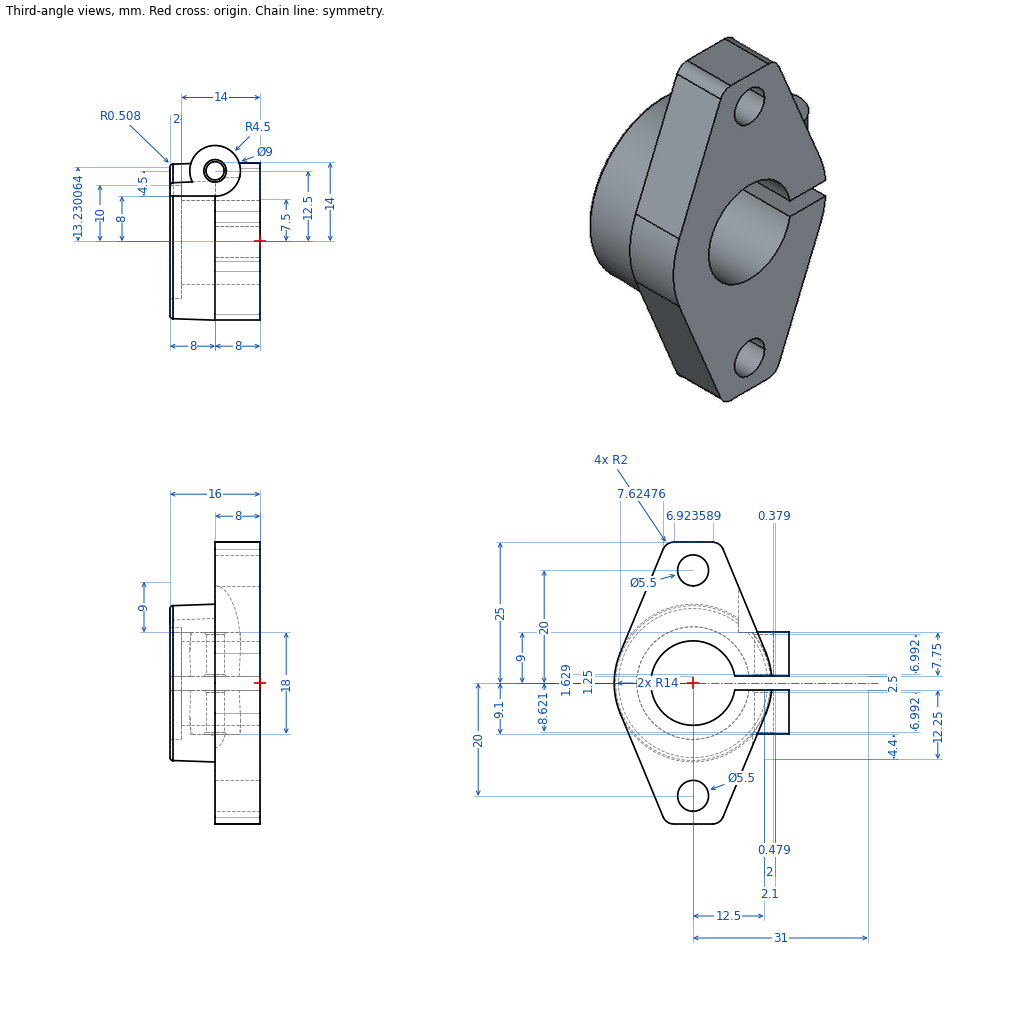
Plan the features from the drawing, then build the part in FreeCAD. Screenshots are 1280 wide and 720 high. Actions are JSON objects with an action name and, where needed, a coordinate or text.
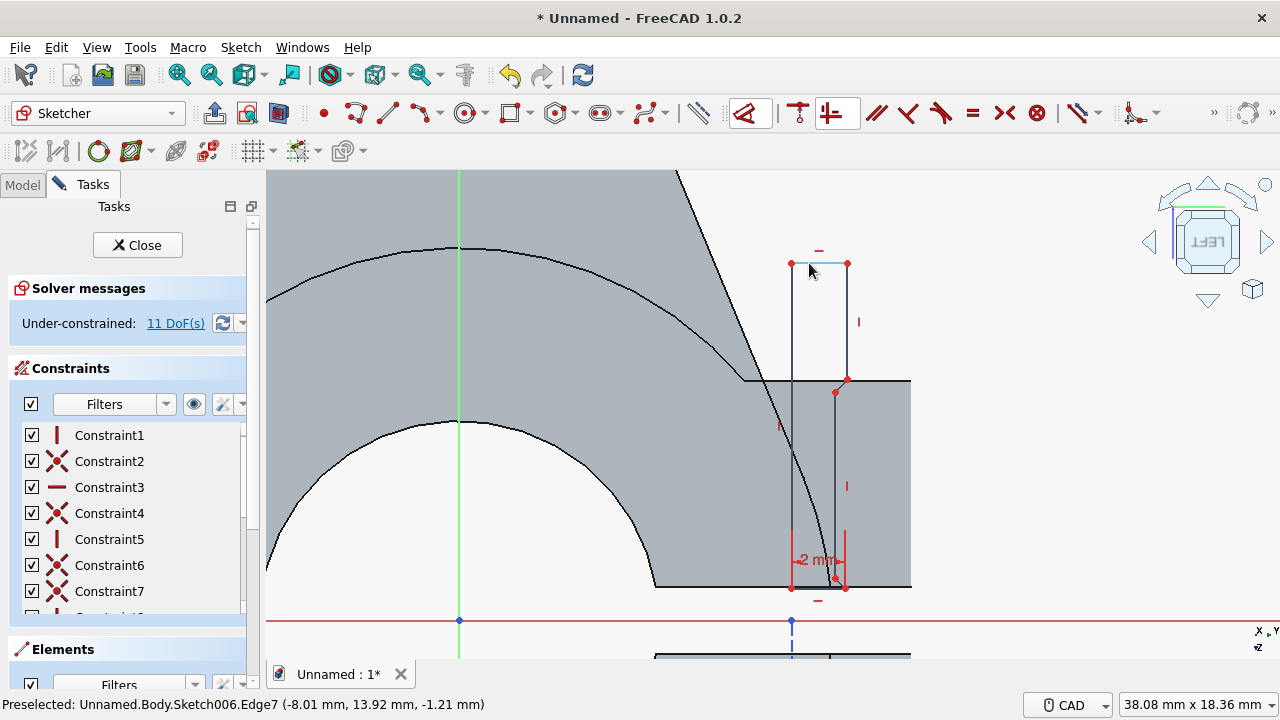
{"action": "left_click", "coordinate": [809, 263]}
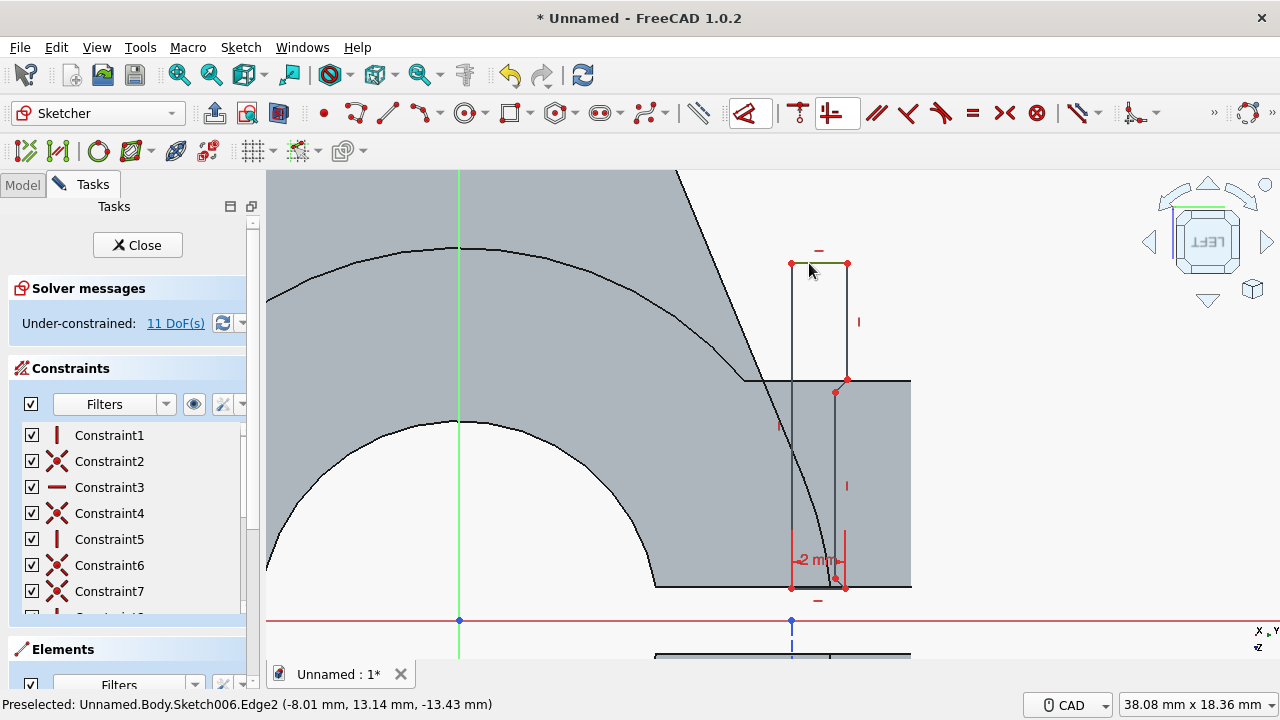
{"action": "key", "text": "l"}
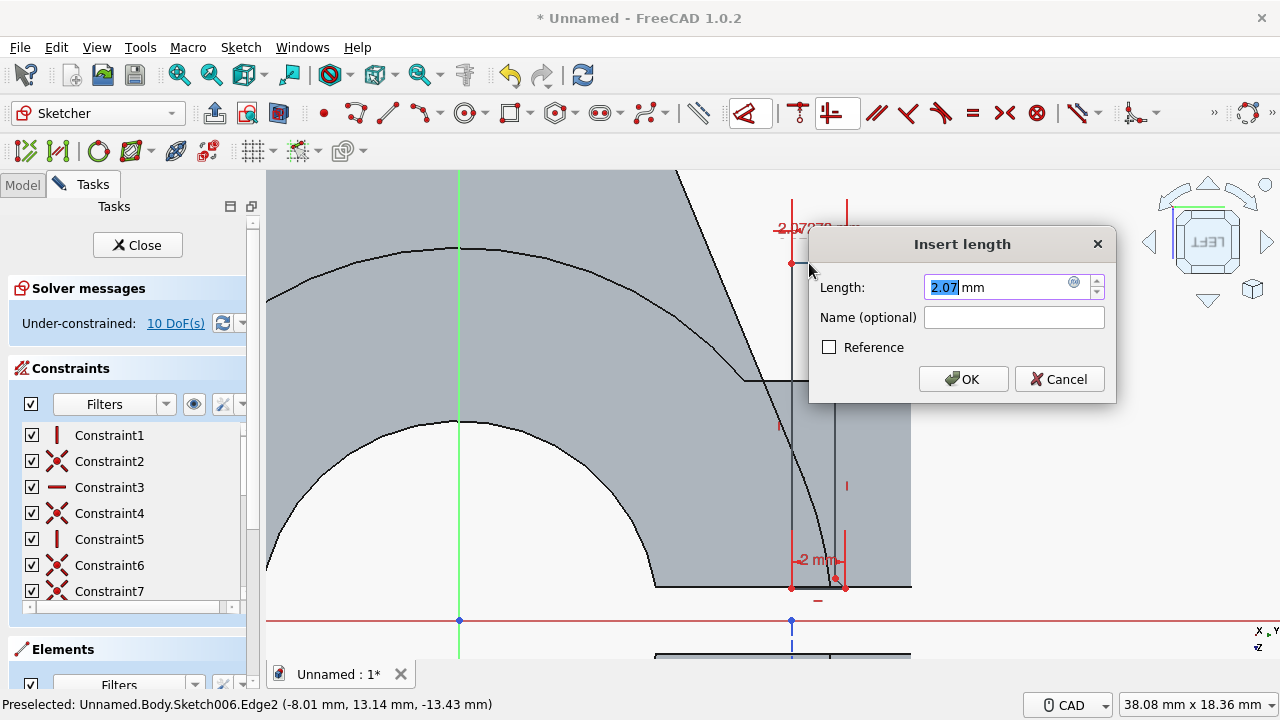
{"action": "type", "text": "2.1"}
{"action": "key", "text": "Return"}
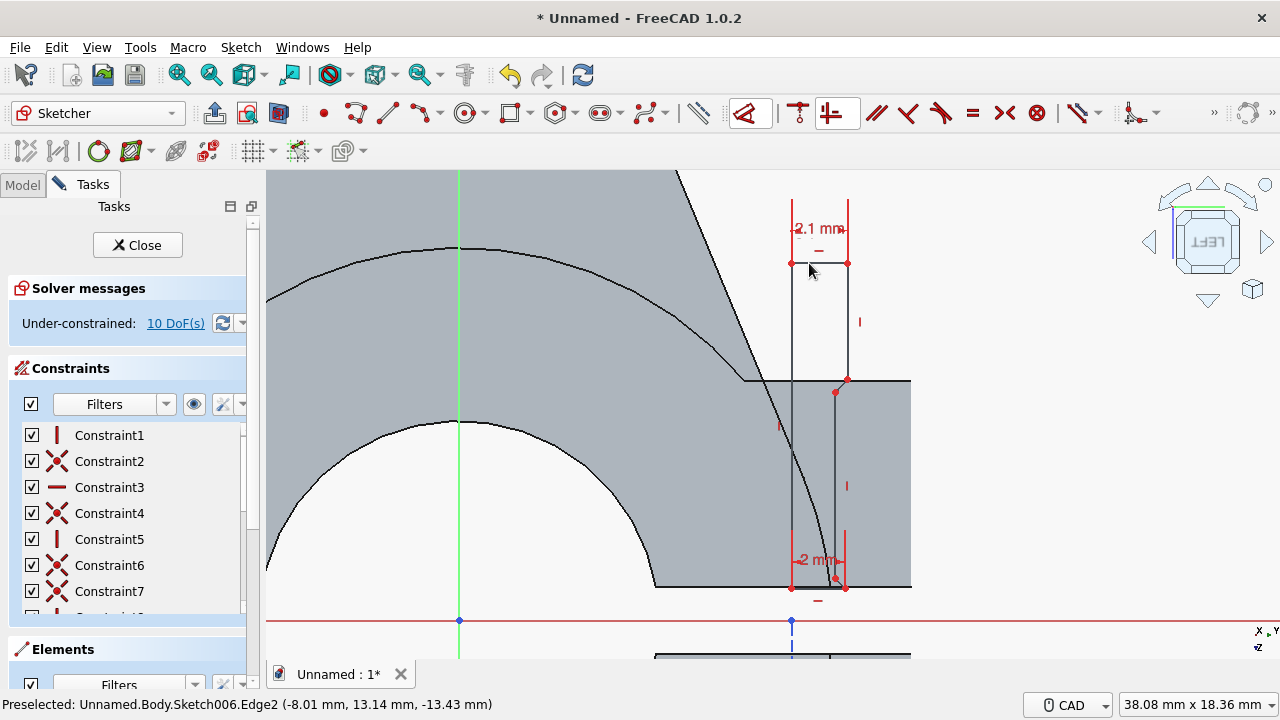
{"action": "left_click", "coordinate": [848, 298]}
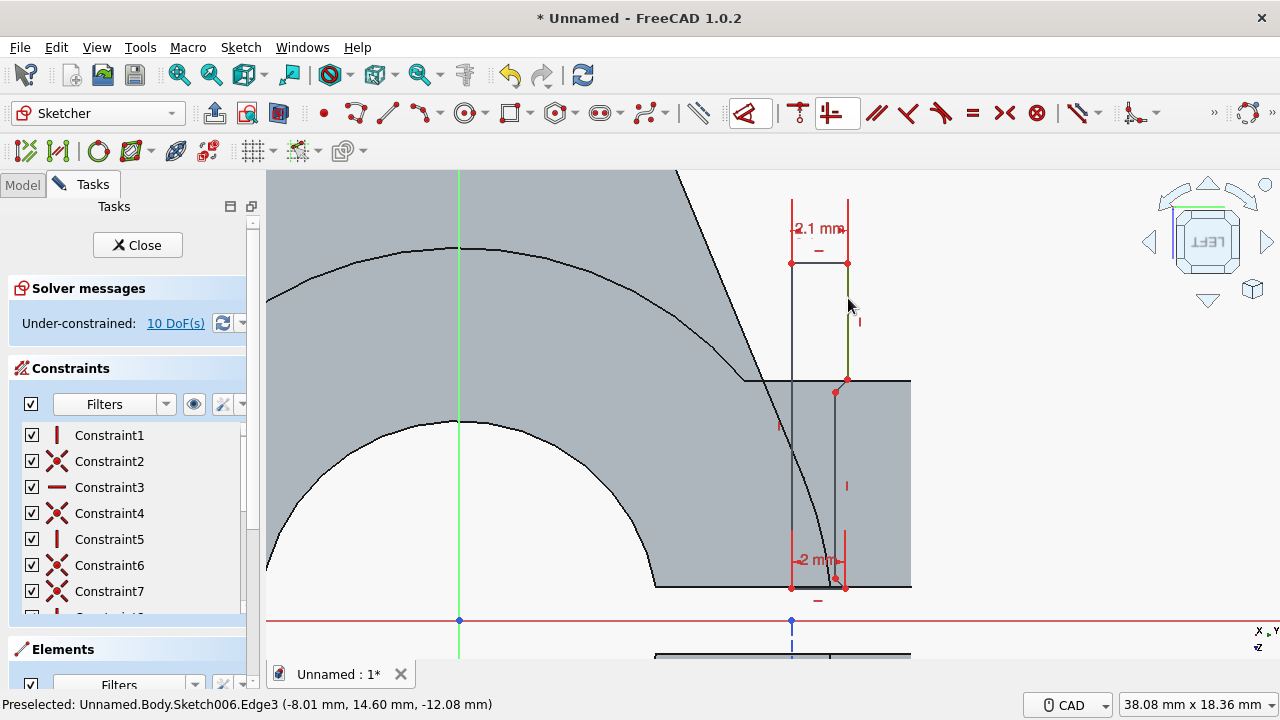
{"action": "key", "text": "i"}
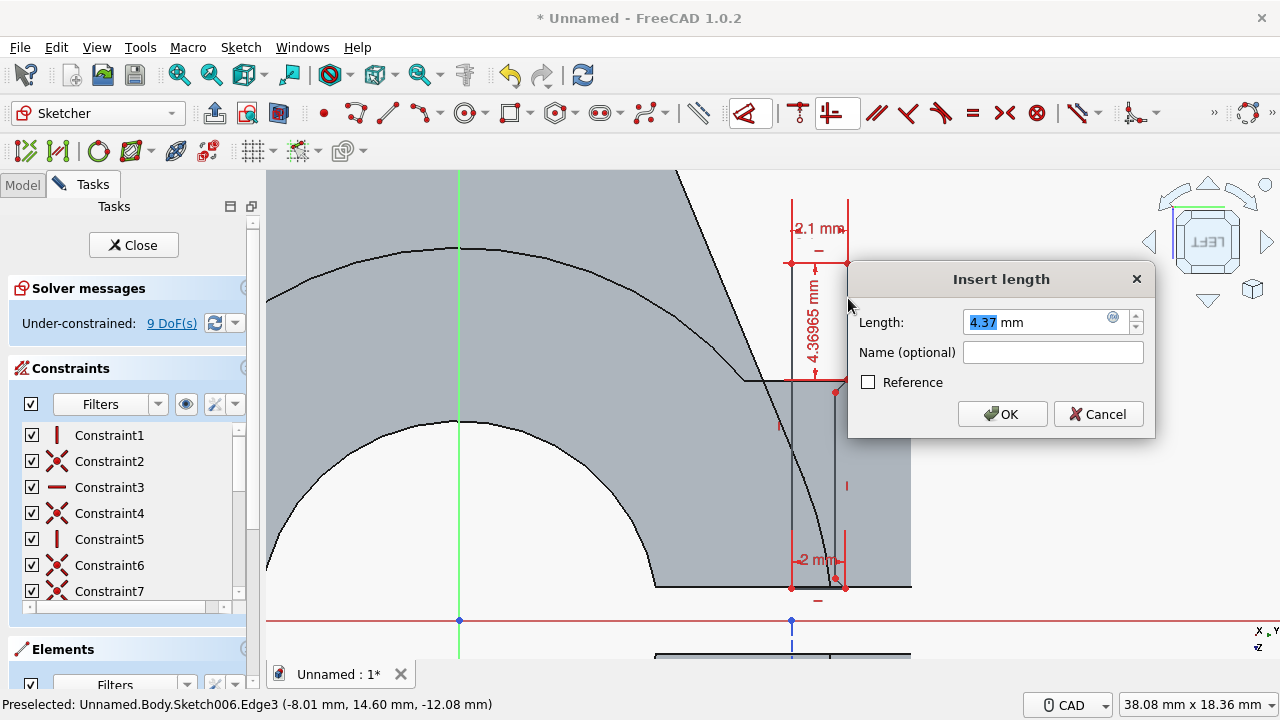
{"action": "type", "text": "4.4"}
{"action": "key", "text": "Return"}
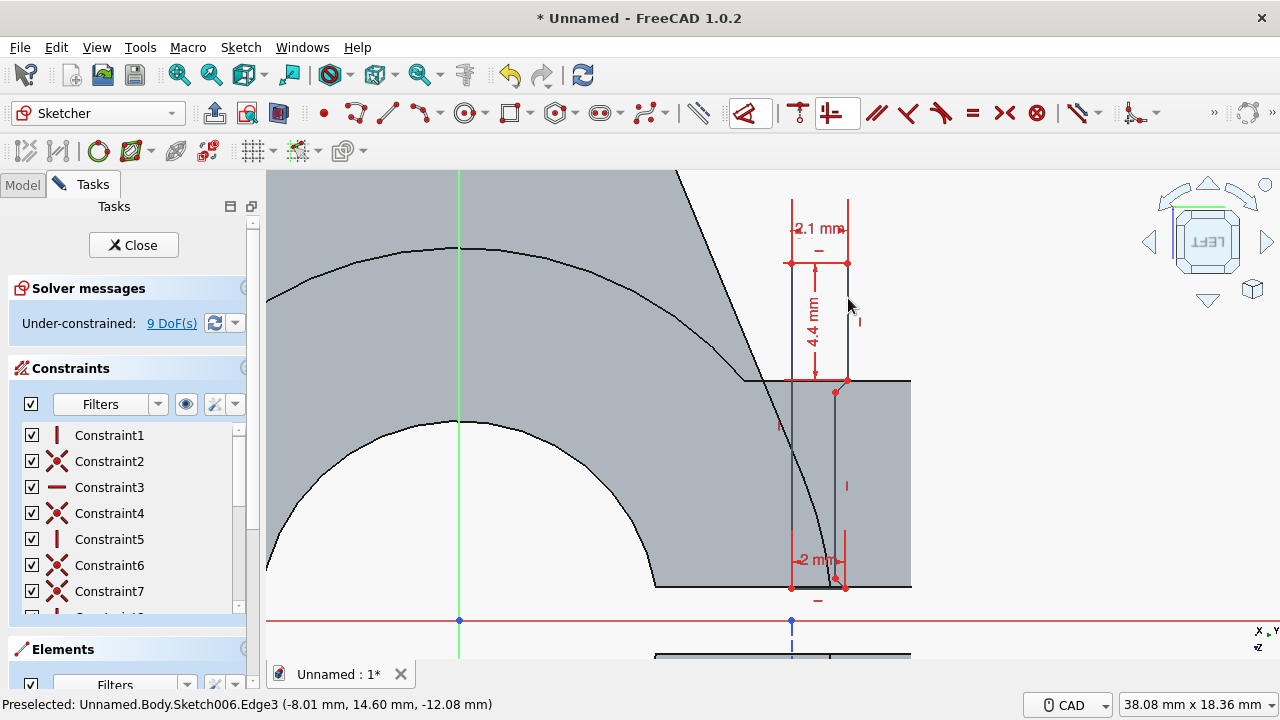
{"action": "left_click", "coordinate": [848, 380]}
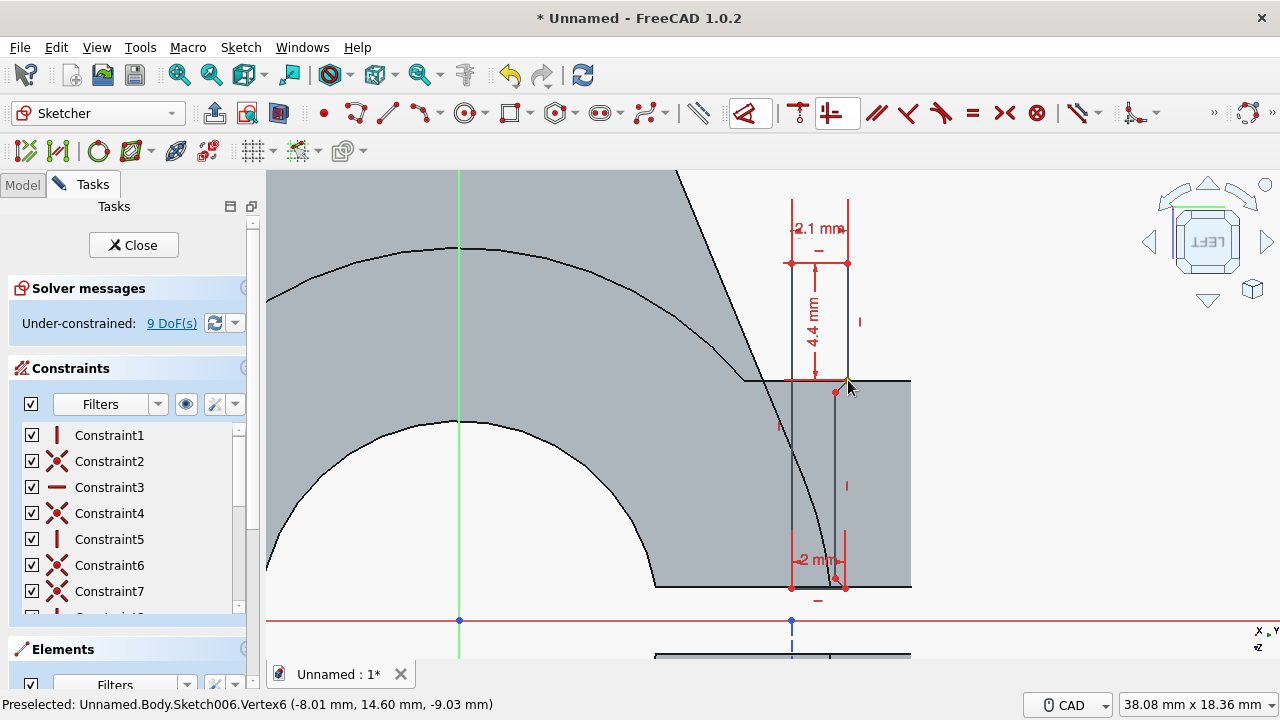
{"action": "left_click", "coordinate": [766, 114]}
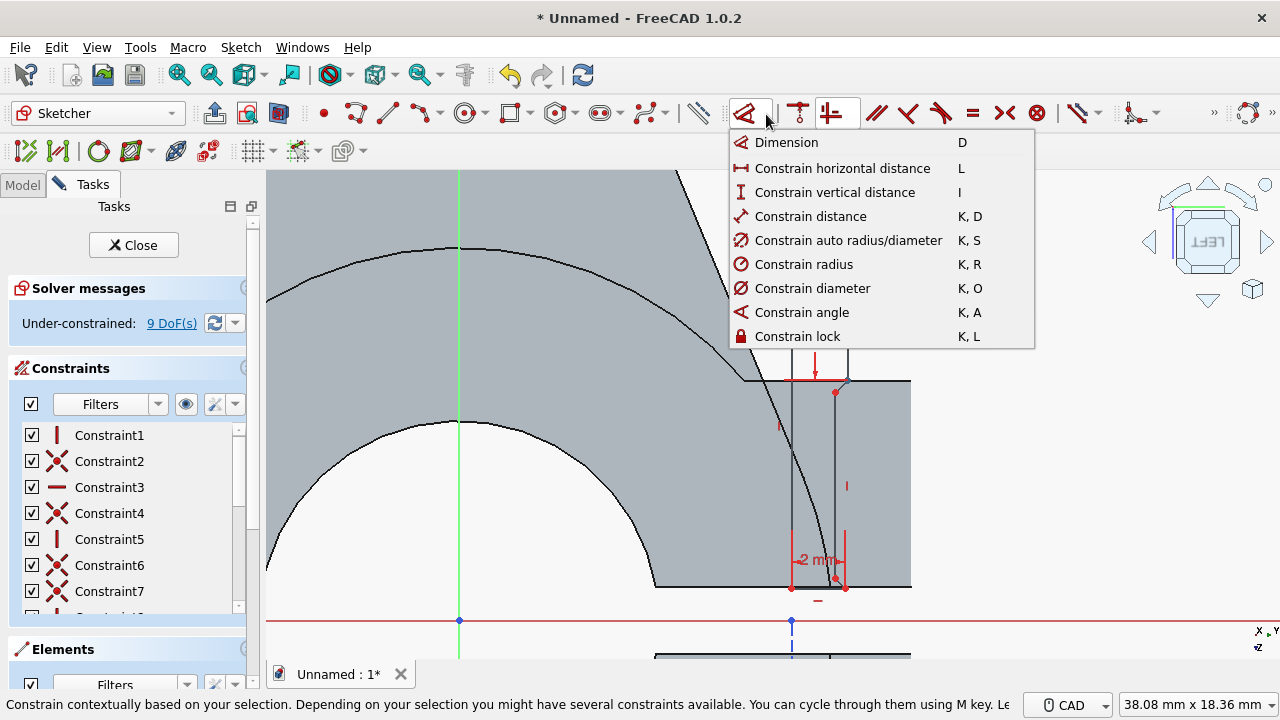
{"action": "left_click", "coordinate": [882, 192]}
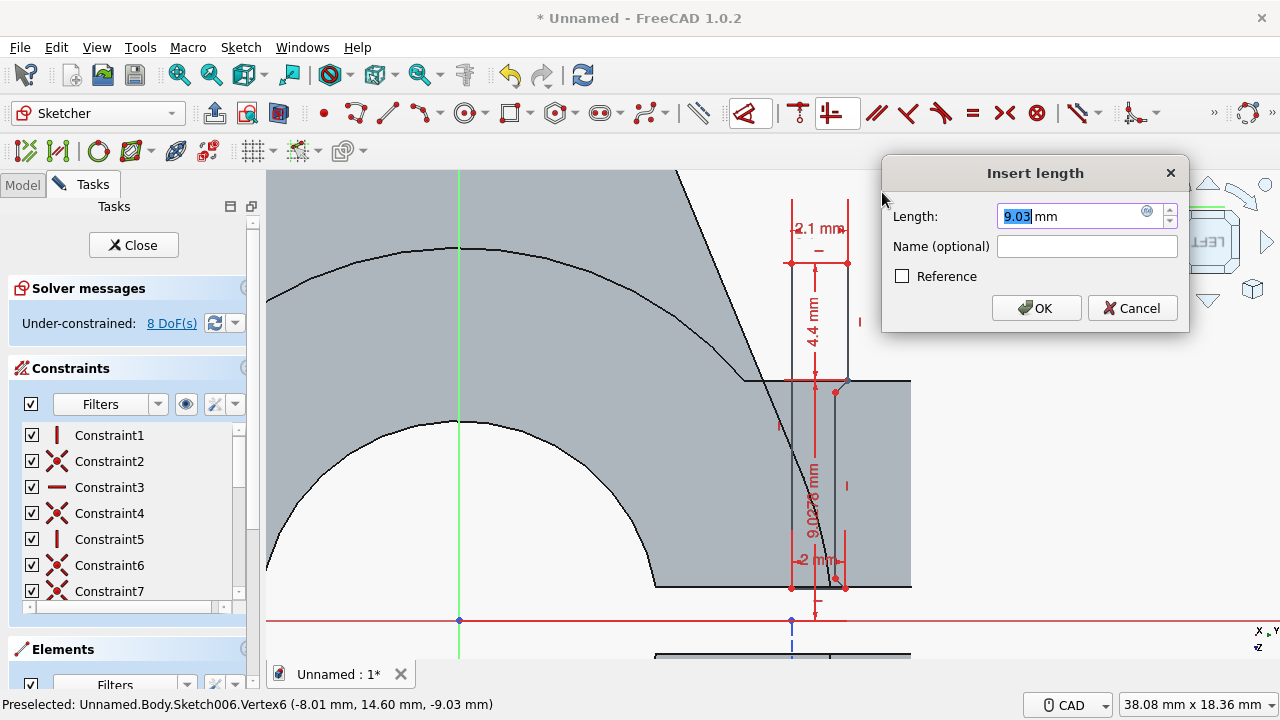
{"action": "type", "text": "9.1"}
{"action": "key", "text": "Return"}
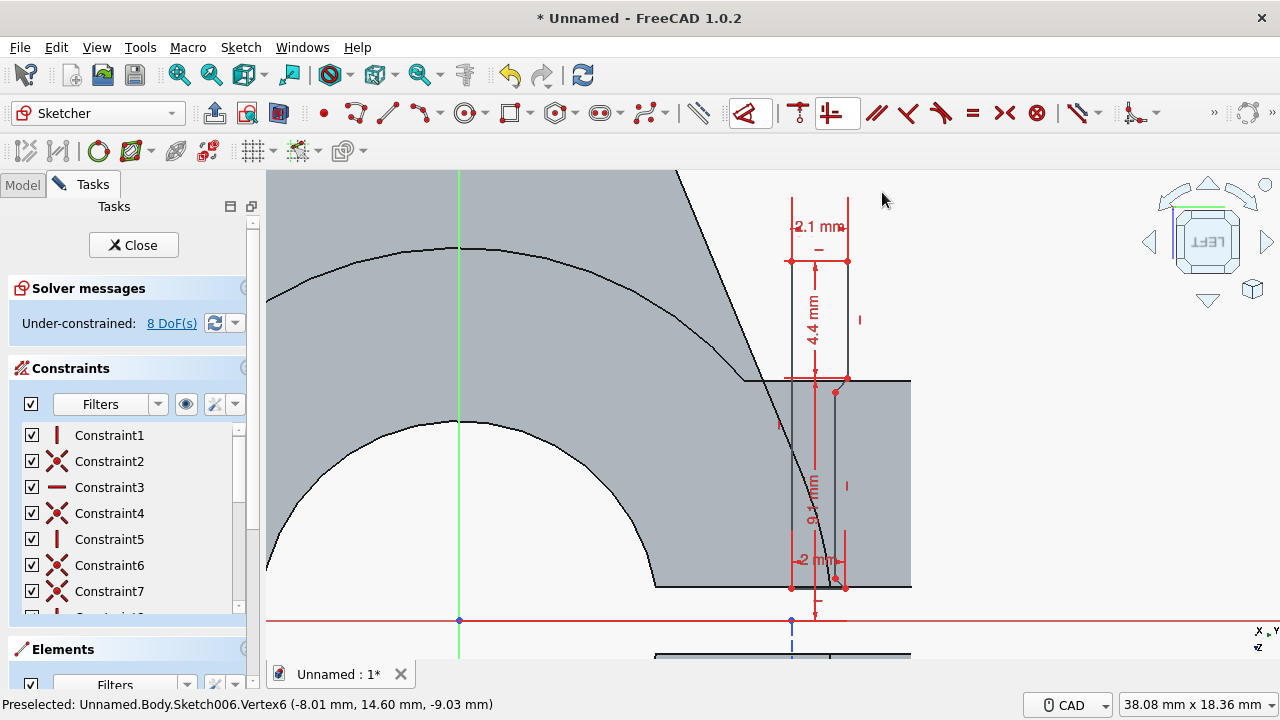
{"action": "left_click", "coordinate": [792, 490]}